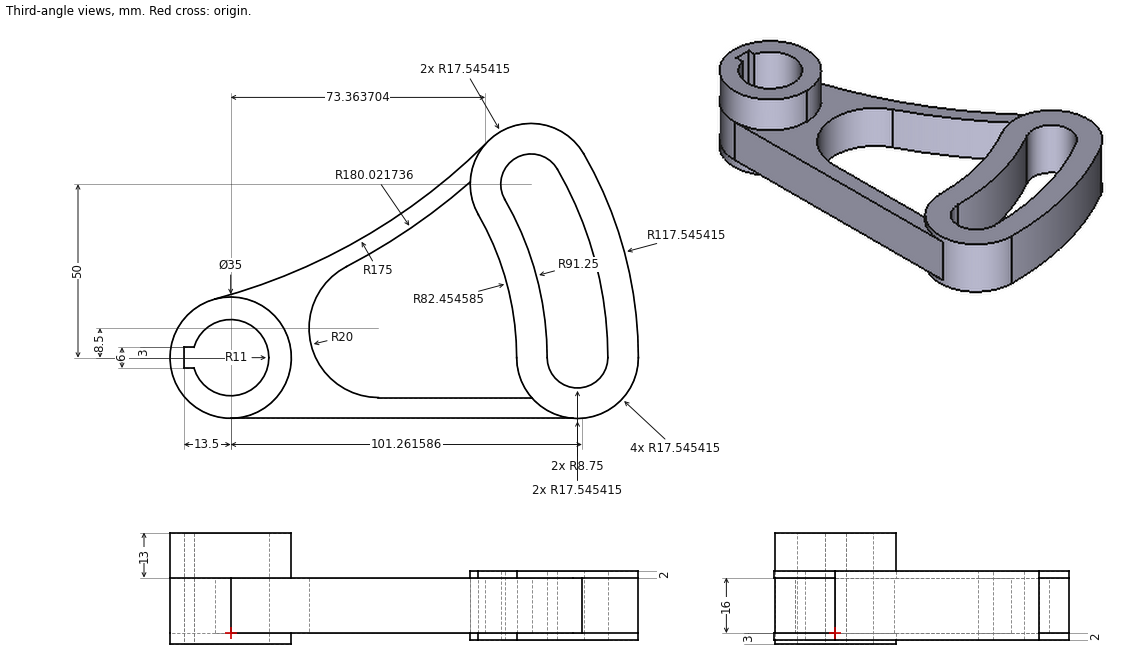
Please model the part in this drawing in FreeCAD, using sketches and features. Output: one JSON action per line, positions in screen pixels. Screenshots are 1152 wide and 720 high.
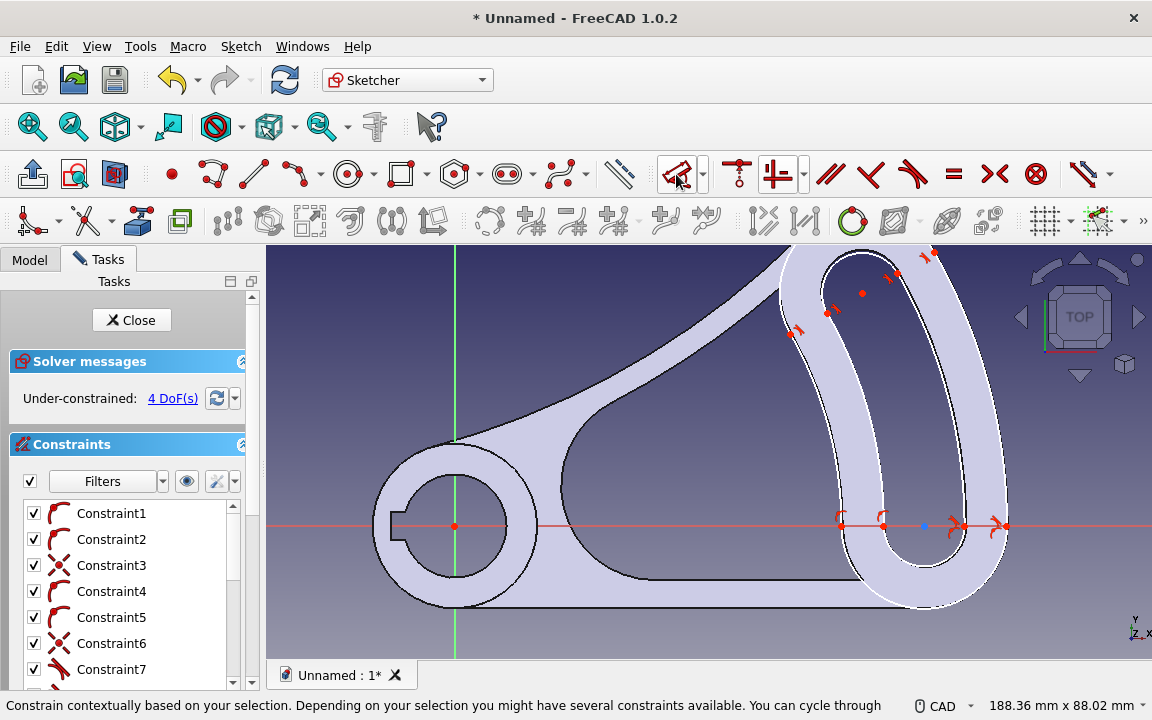
{"action": "left_click", "coordinate": [876, 593]}
{"action": "left_click", "coordinate": [857, 619]}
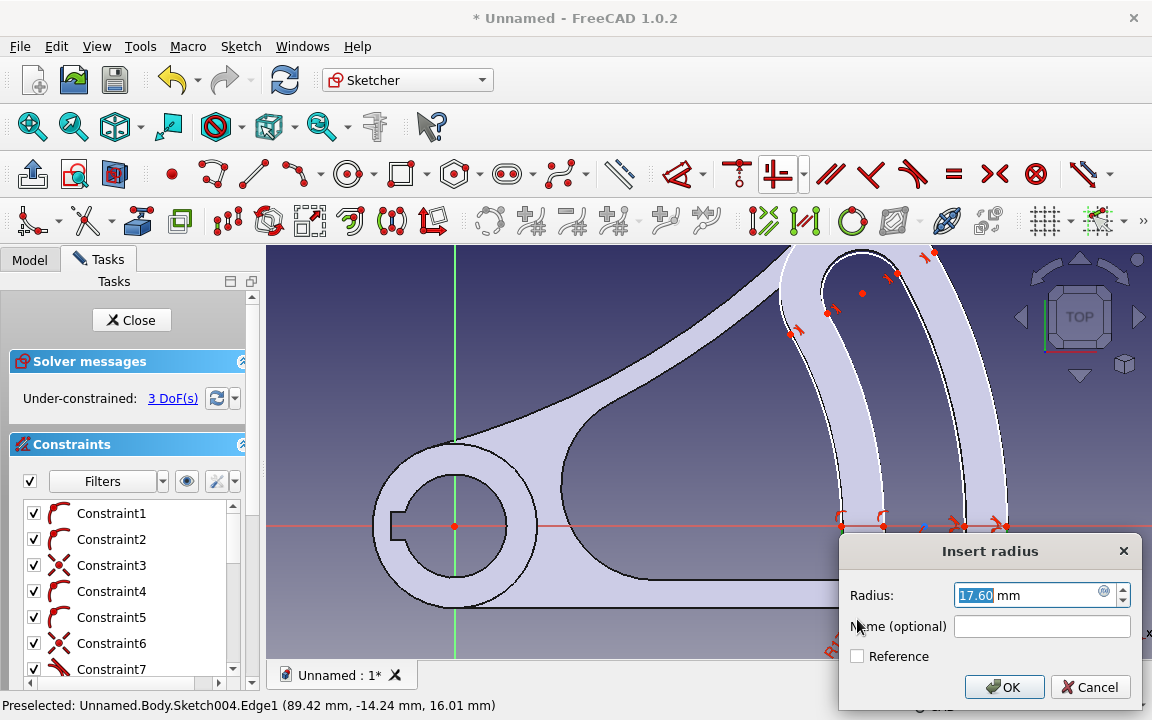
{"action": "type", "text": "17.545415"}
{"action": "key", "text": "Return"}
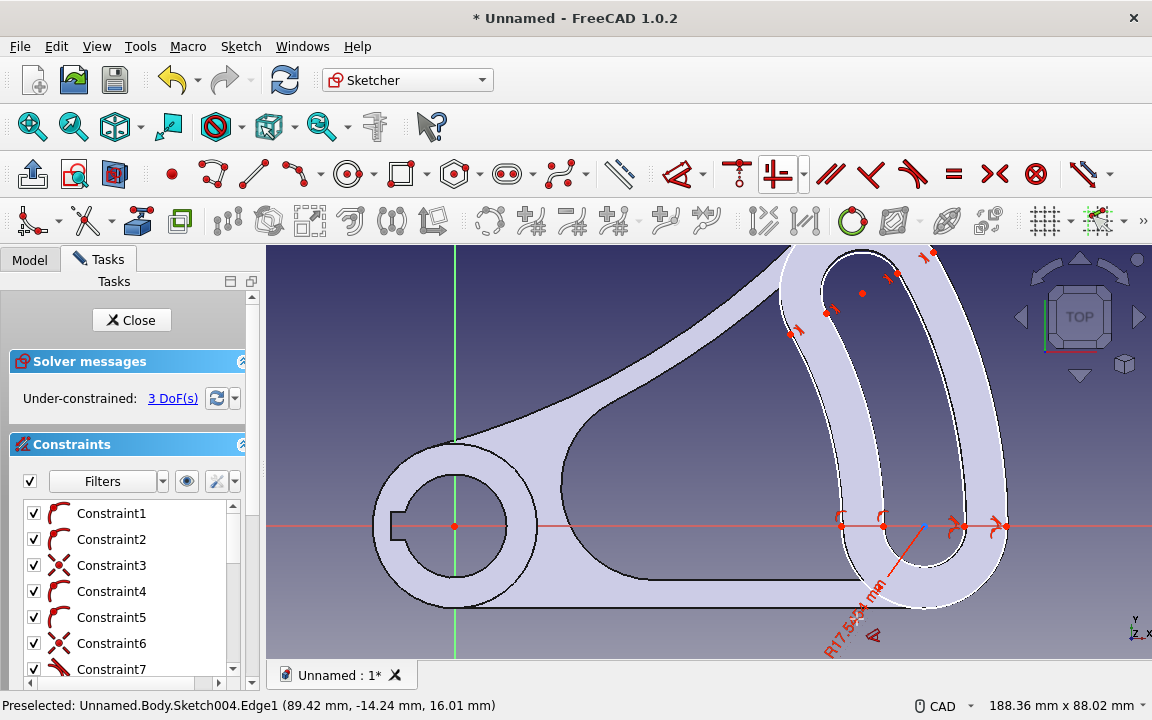
{"action": "left_click", "coordinate": [971, 330]}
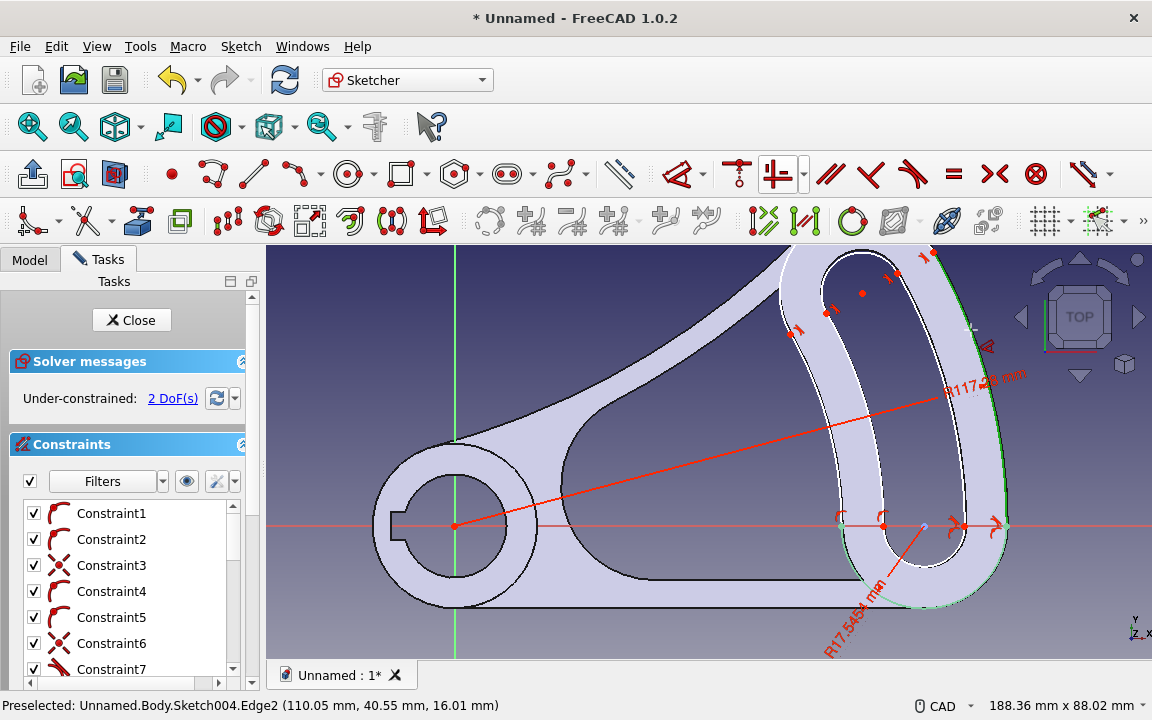
{"action": "key", "text": "Escape"}
{"action": "key", "text": "Escape"}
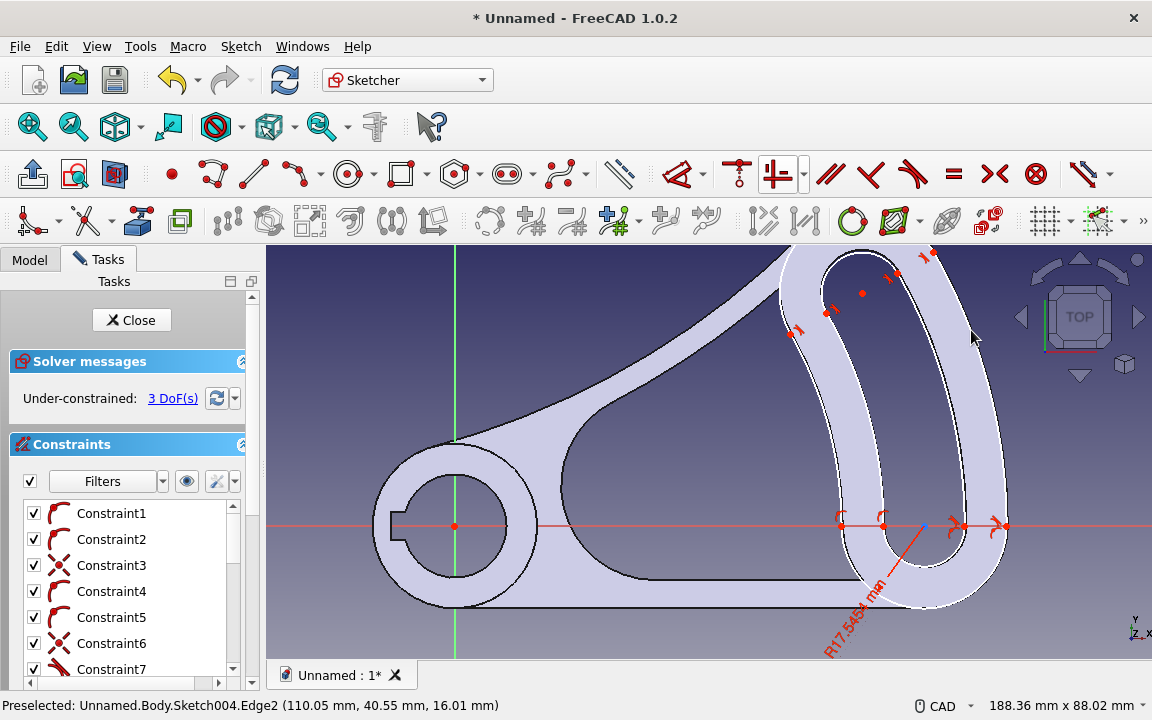
{"action": "left_click", "coordinate": [971, 330]}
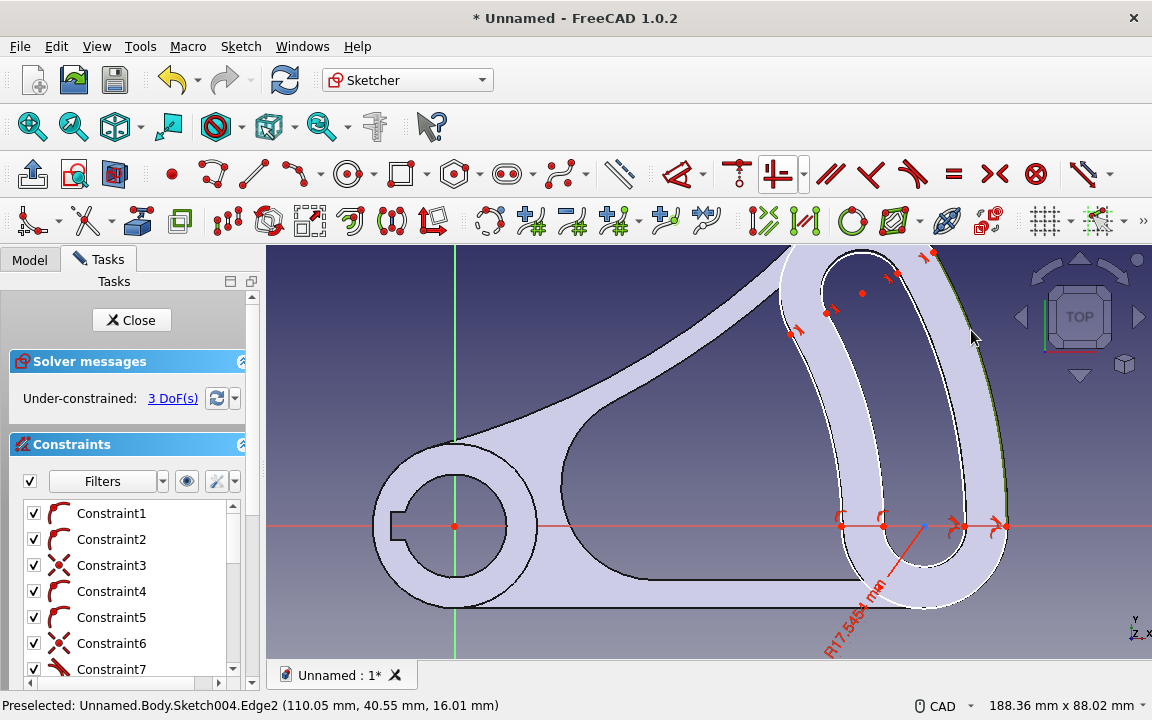
{"action": "key", "text": "k r"}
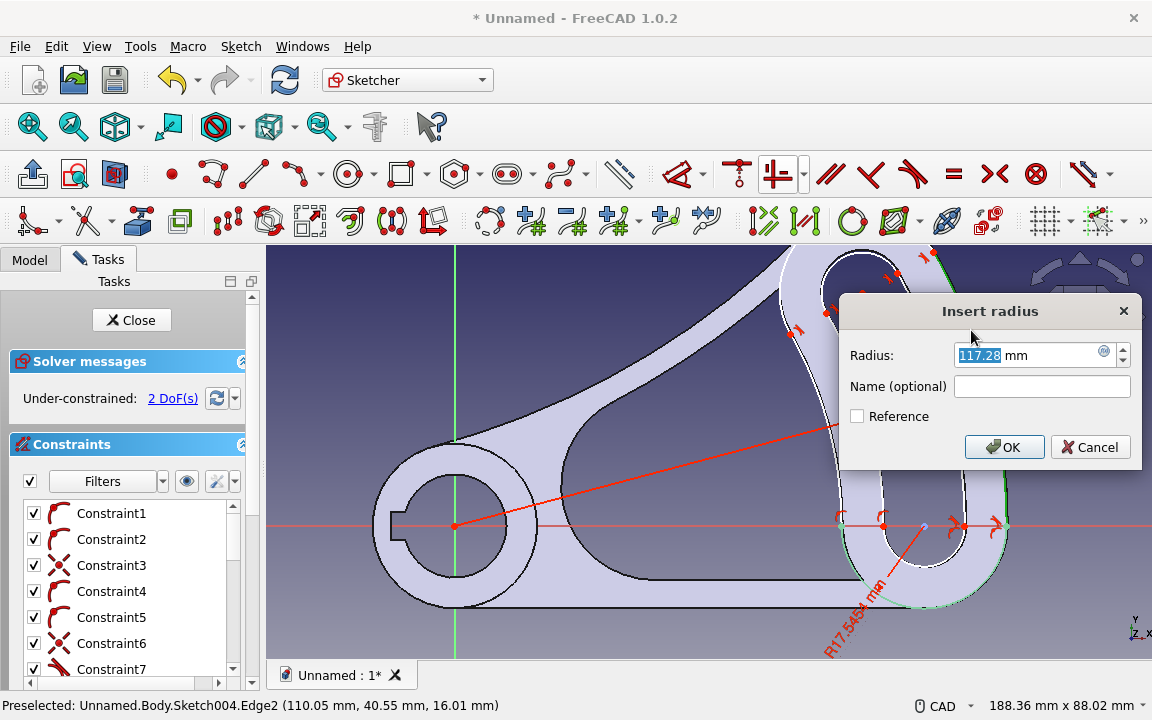
{"action": "type", "text": "117.545415"}
{"action": "key", "text": "Return"}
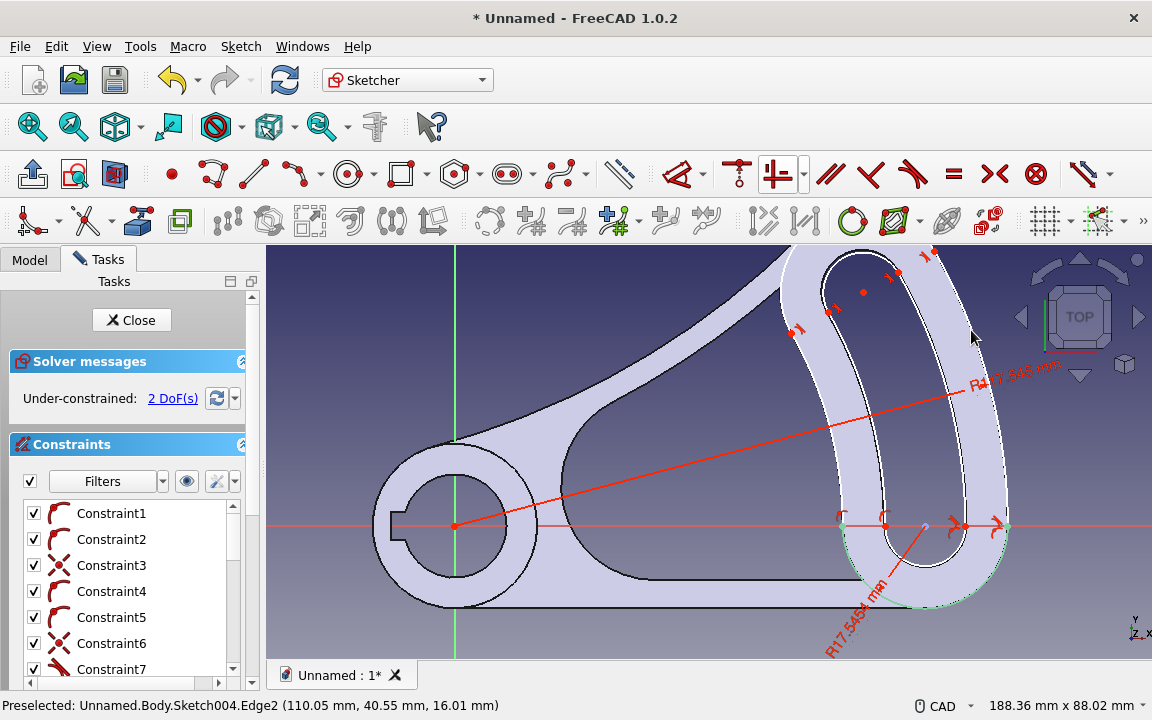
{"action": "left_click", "coordinate": [827, 276]}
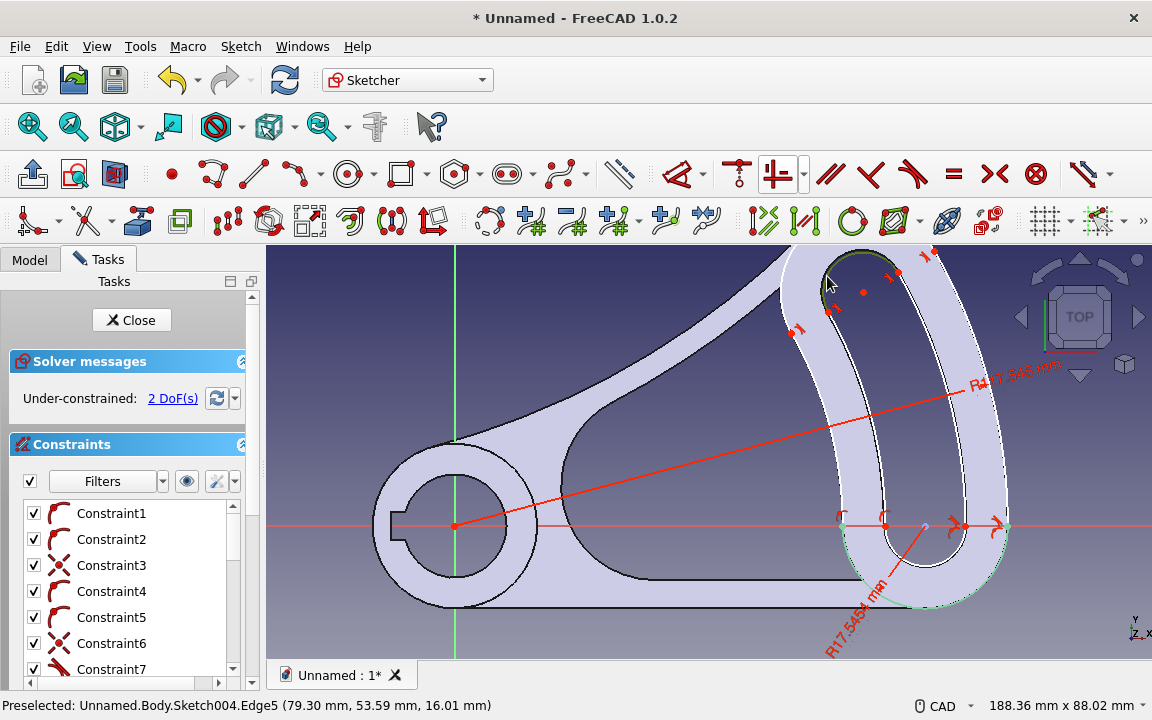
{"action": "left_click", "coordinate": [702, 174]}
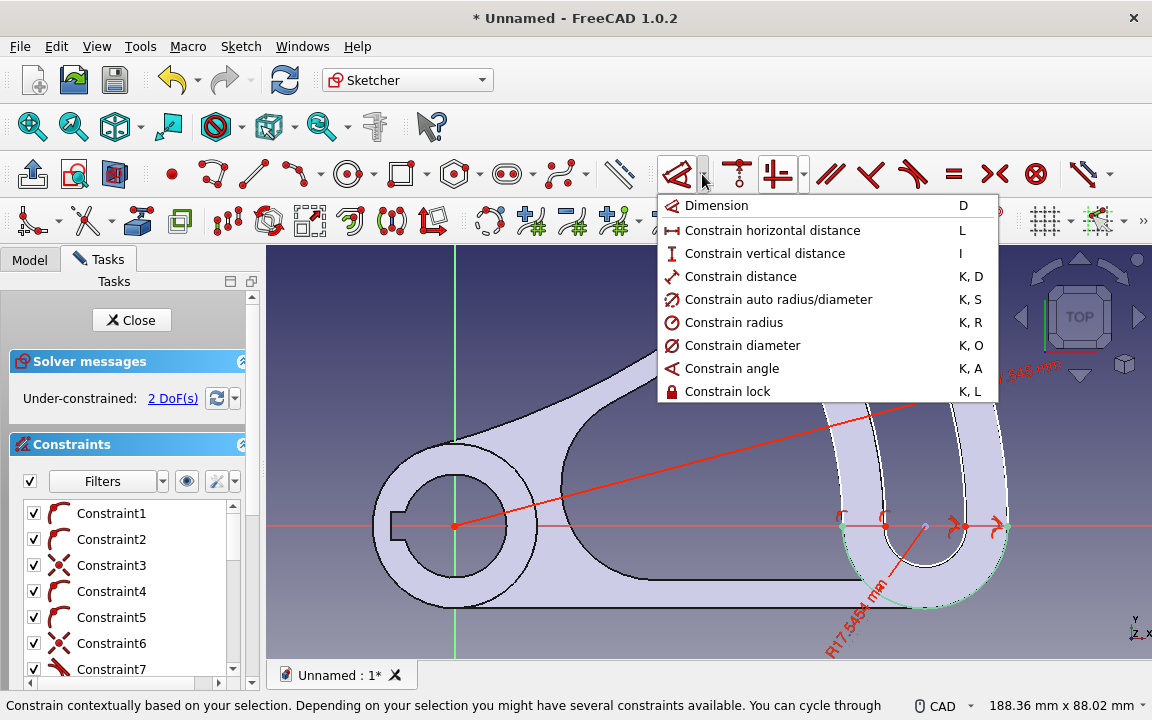
{"action": "left_click", "coordinate": [828, 322]}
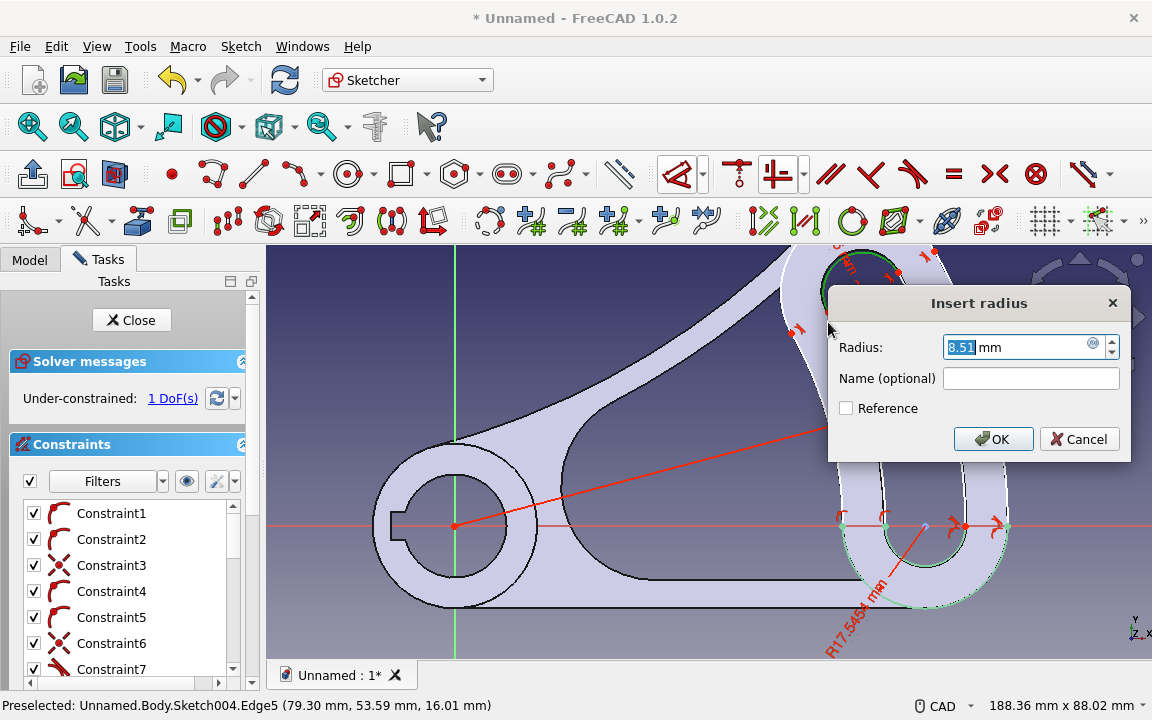
{"action": "type", "text": "8.75"}
{"action": "key", "text": "Return"}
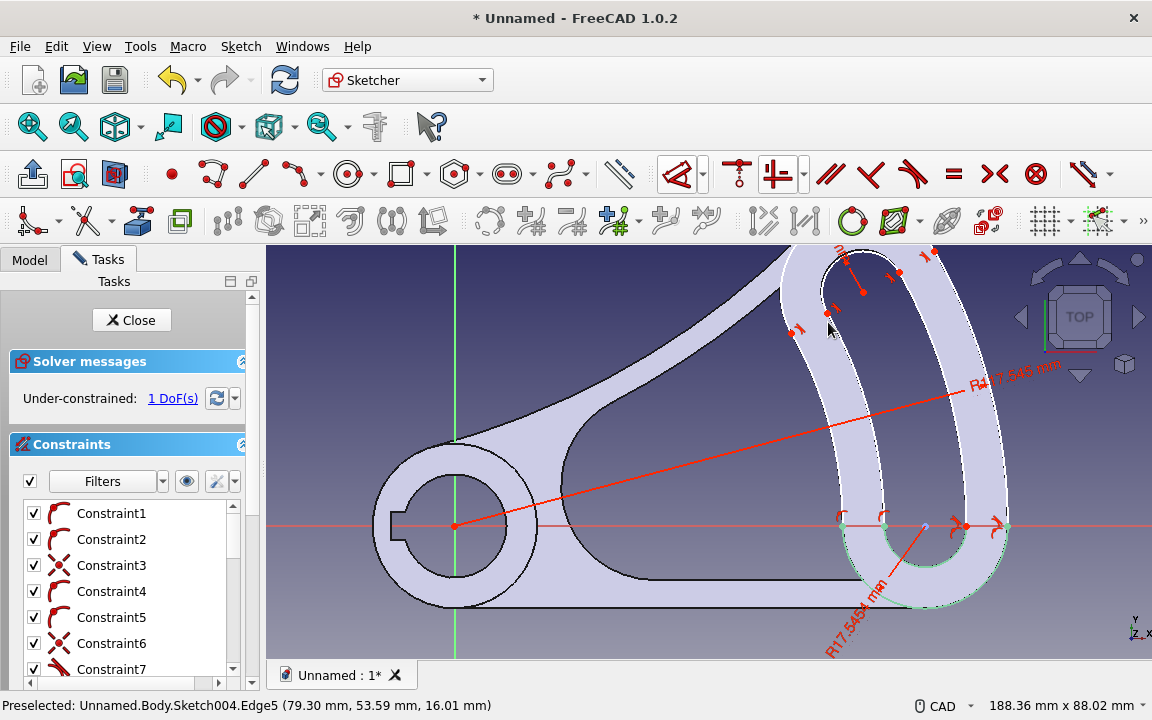
{"action": "left_click", "coordinate": [863, 293]}